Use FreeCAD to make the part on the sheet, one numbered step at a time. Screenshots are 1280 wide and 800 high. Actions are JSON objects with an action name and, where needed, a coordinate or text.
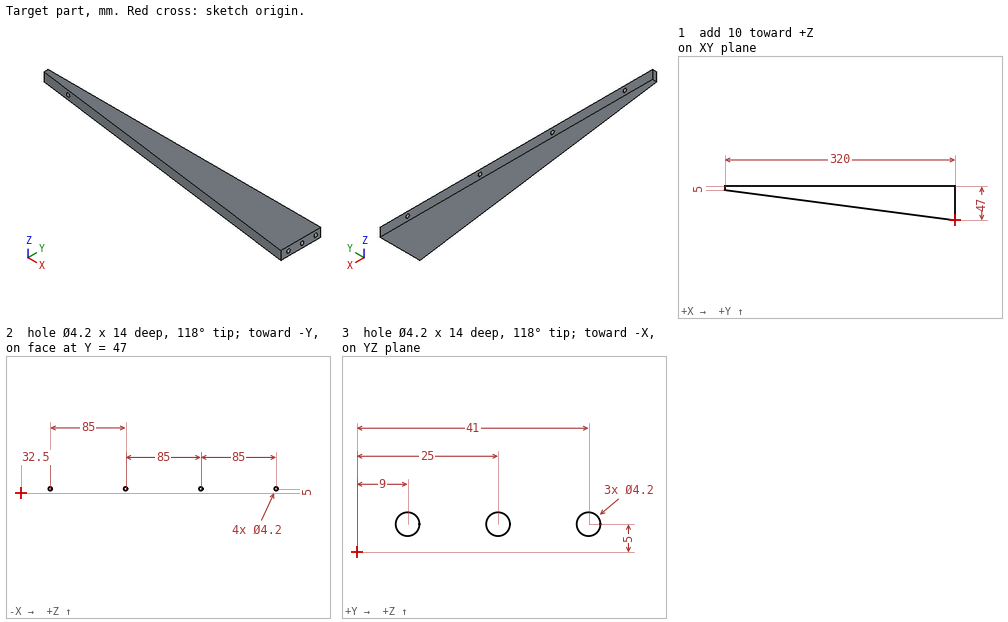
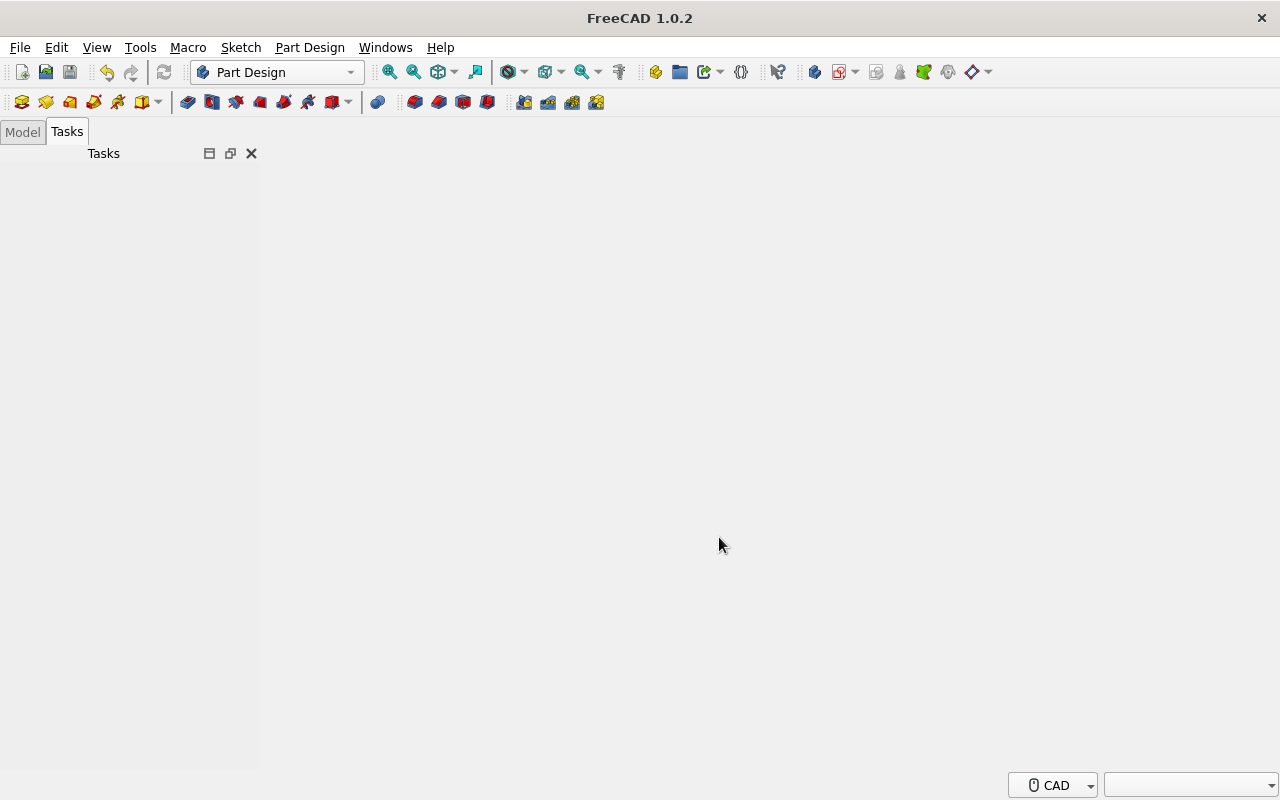
{"action": "key", "text": "ctrl+n"}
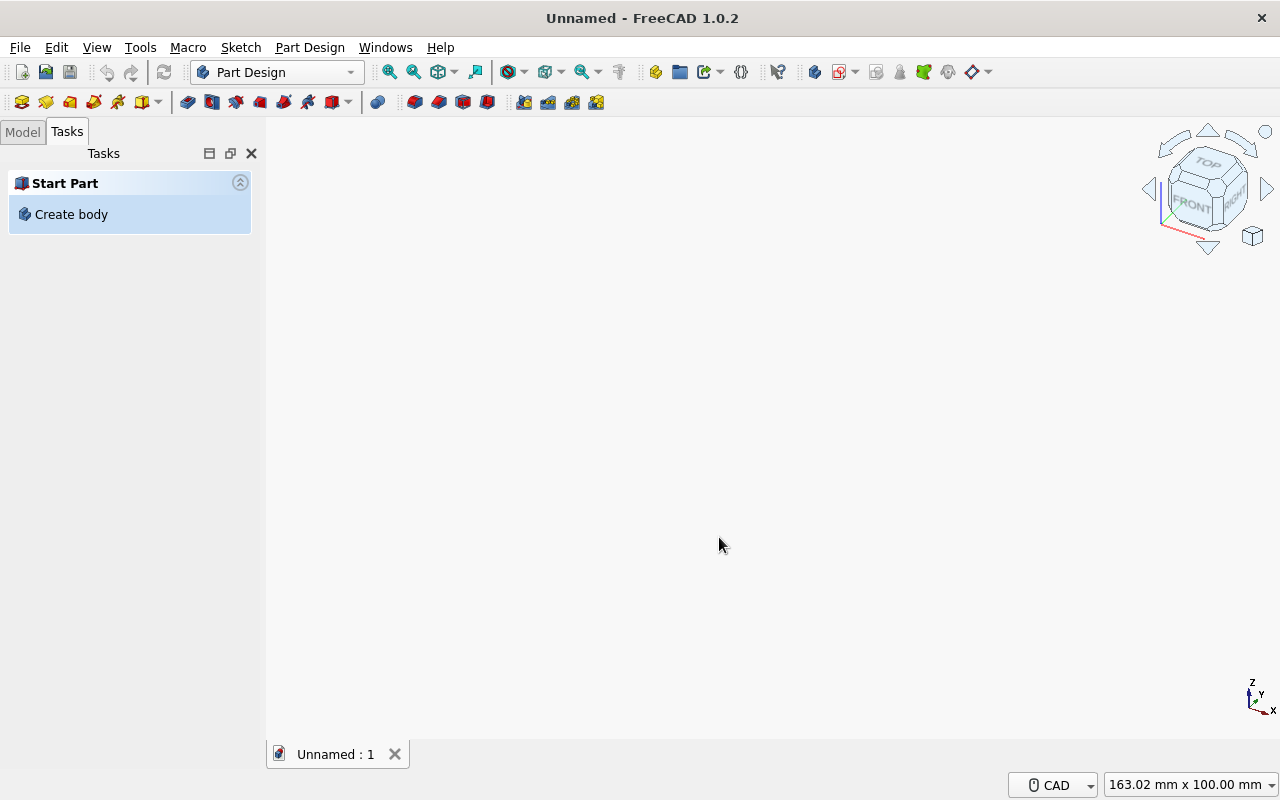
{"action": "left_click", "coordinate": [840, 72]}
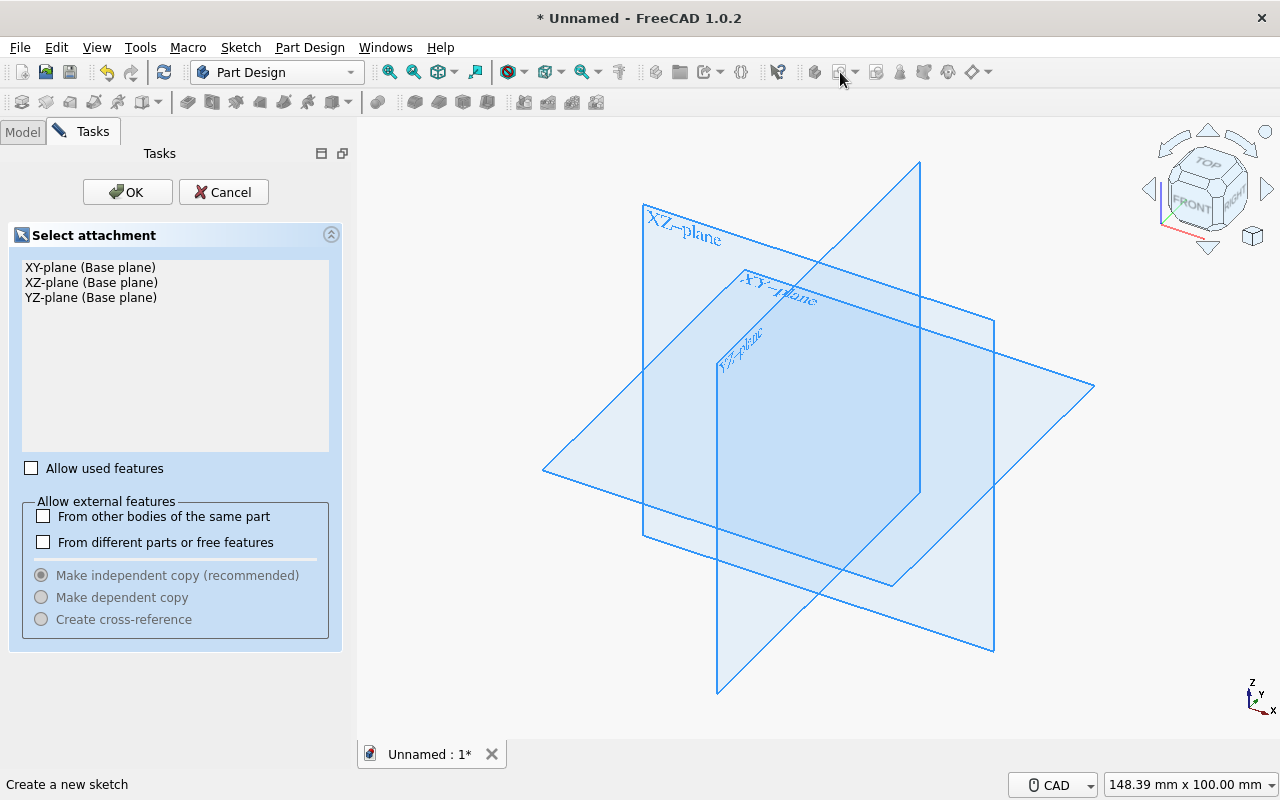
{"action": "left_click", "coordinate": [82, 268]}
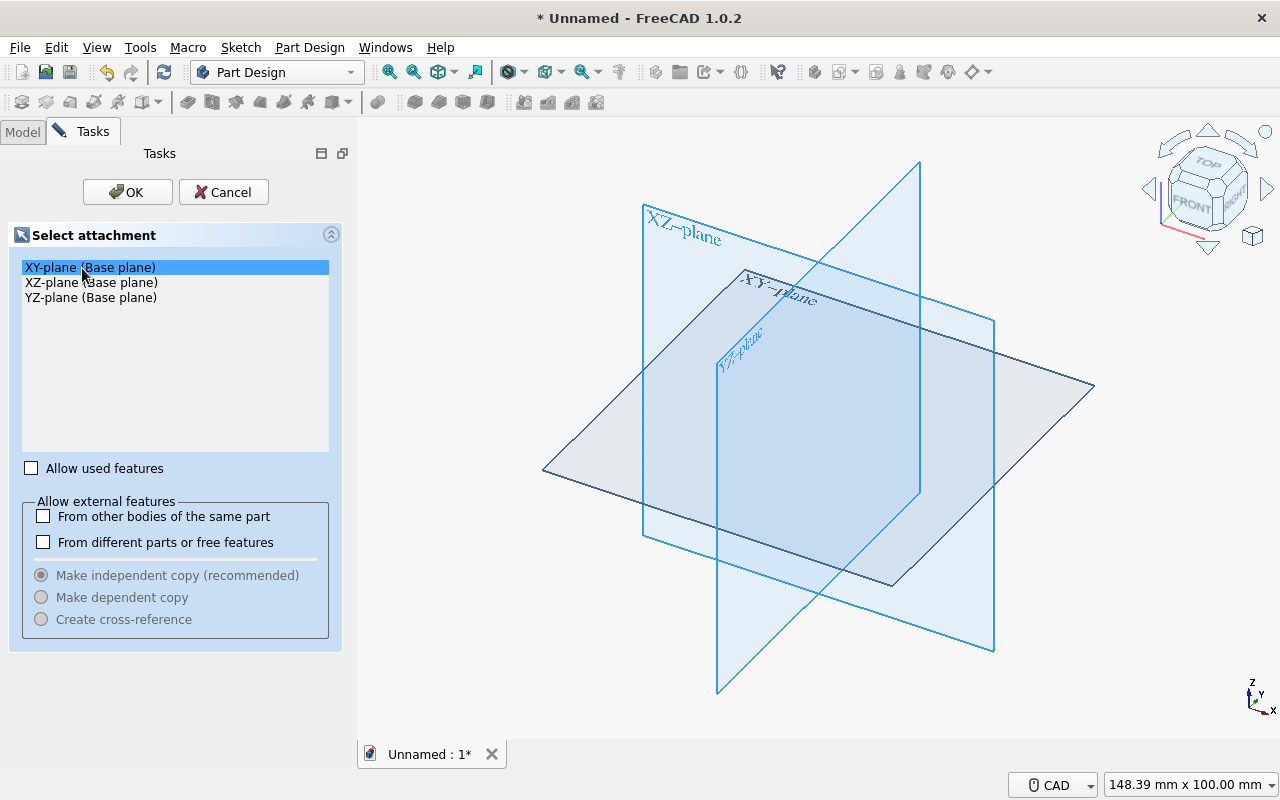
{"action": "left_click", "coordinate": [128, 192]}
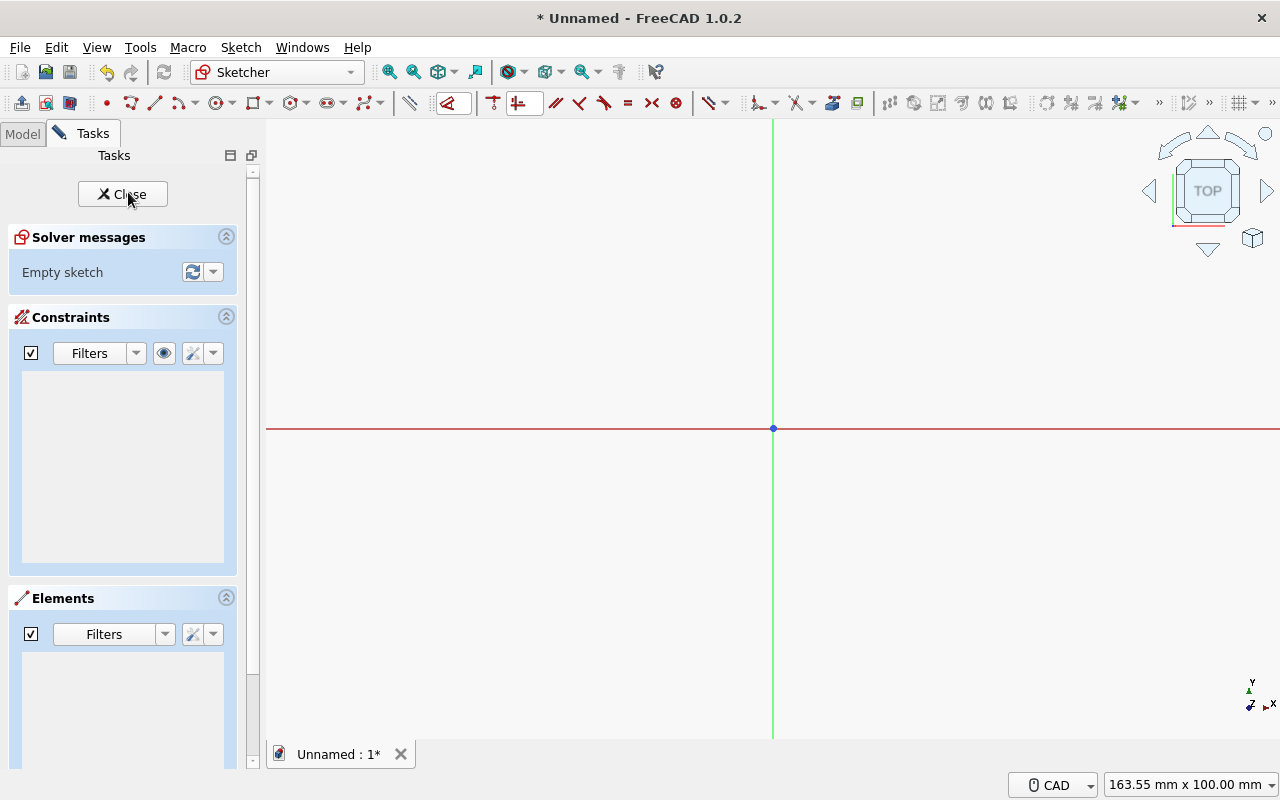
{"action": "scroll", "coordinate": [1103, 492], "scroll_direction": "down", "scroll_amount": 6}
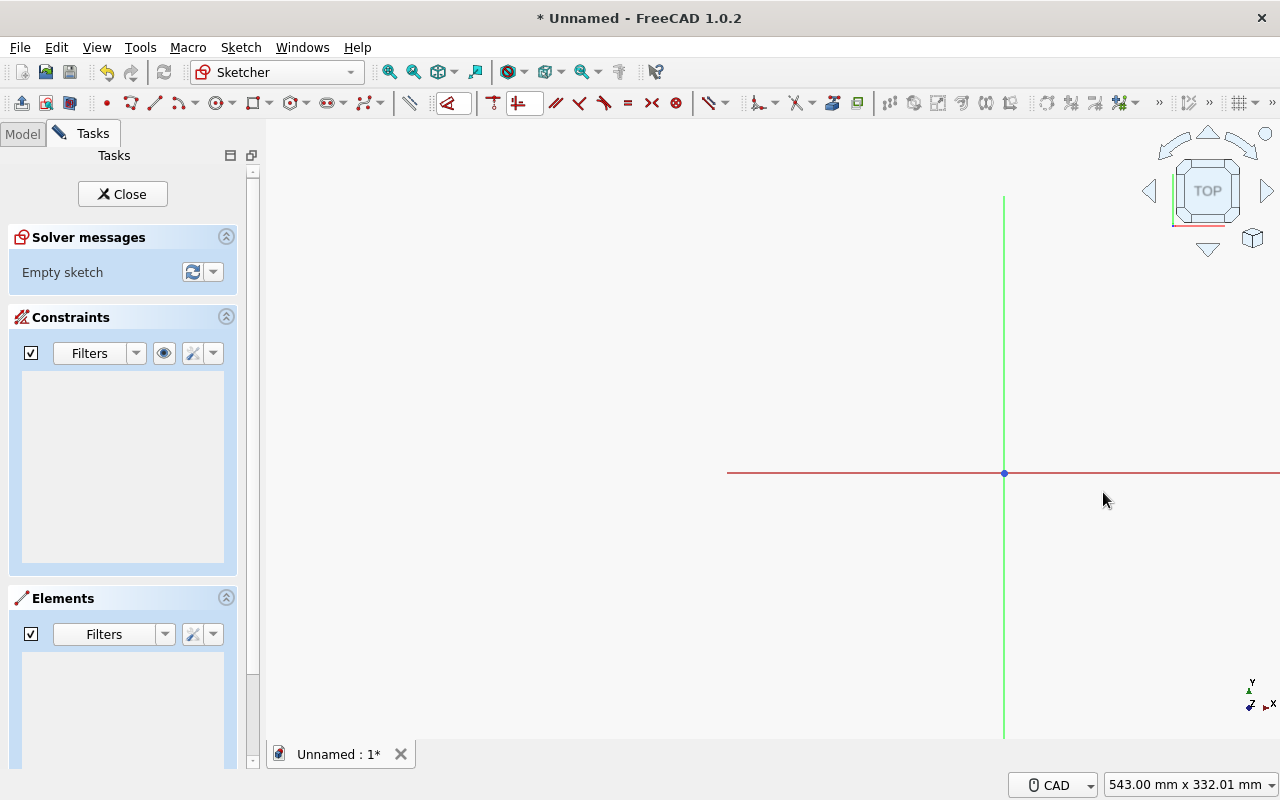
{"action": "left_click", "coordinate": [132, 104]}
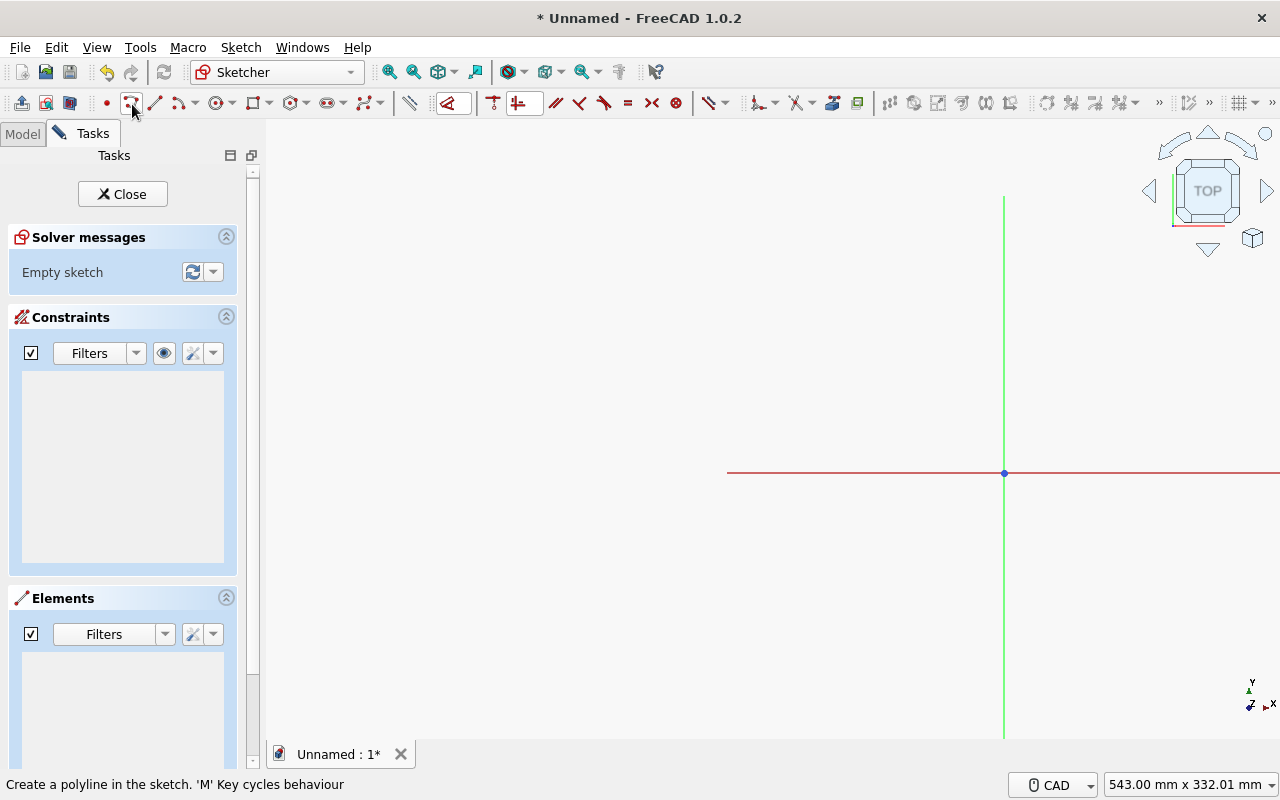
{"action": "left_click", "coordinate": [1004, 473]}
{"action": "left_click", "coordinate": [995, 386]}
{"action": "left_click", "coordinate": [407, 386]}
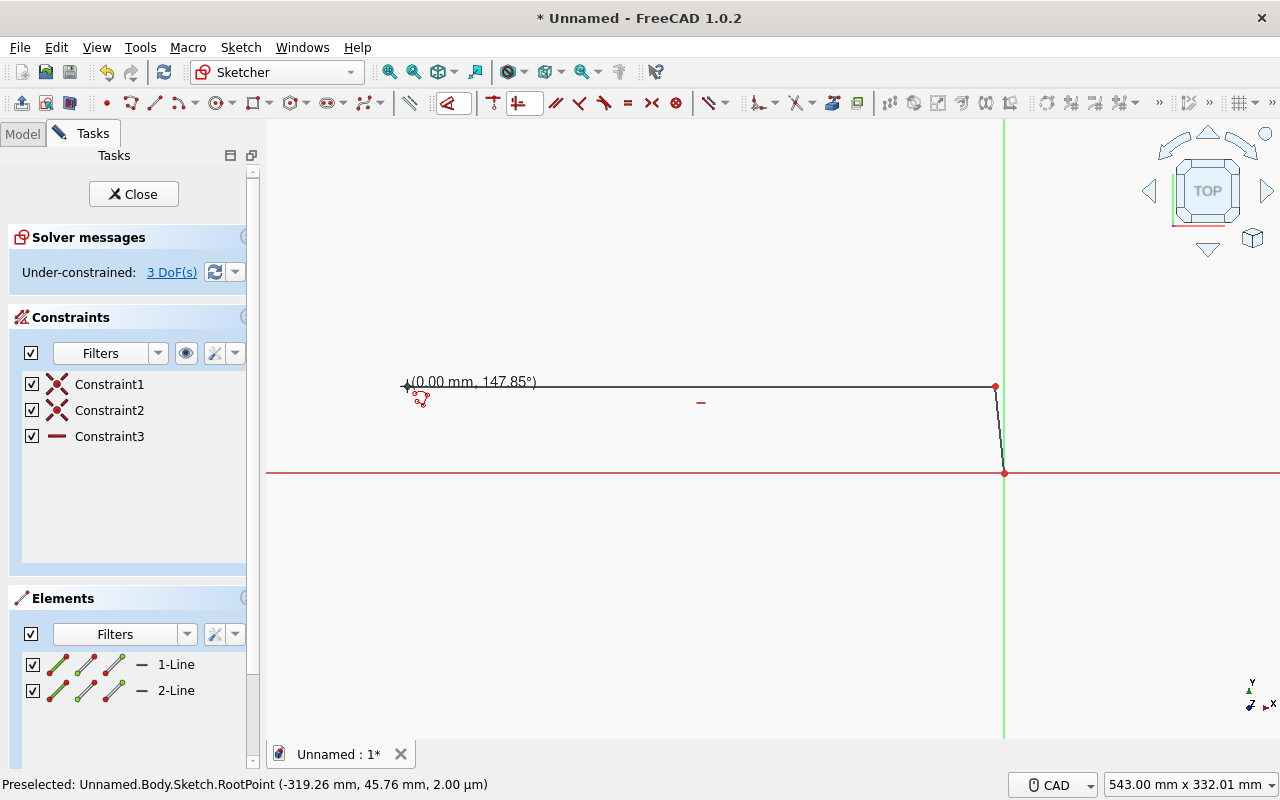
{"action": "scroll", "coordinate": [407, 395], "scroll_direction": "up", "scroll_amount": 3}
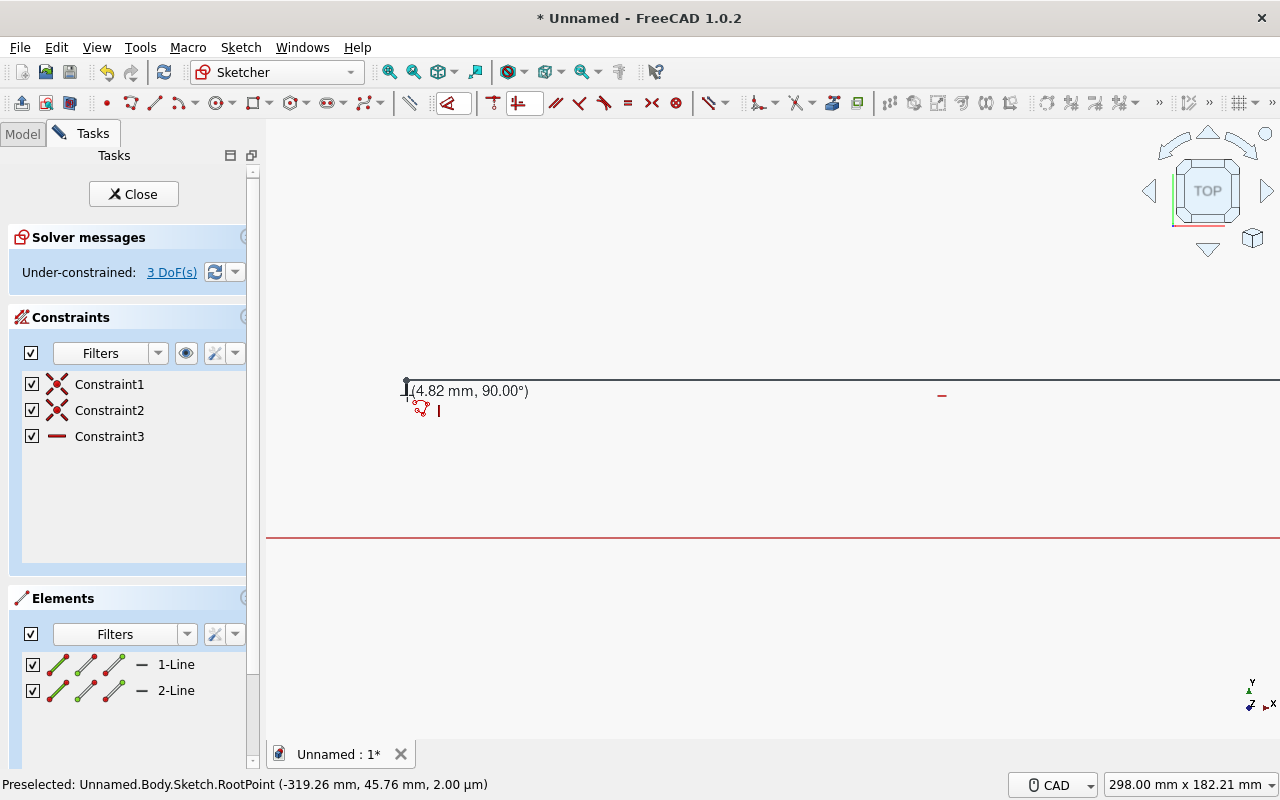
{"action": "left_click", "coordinate": [407, 395]}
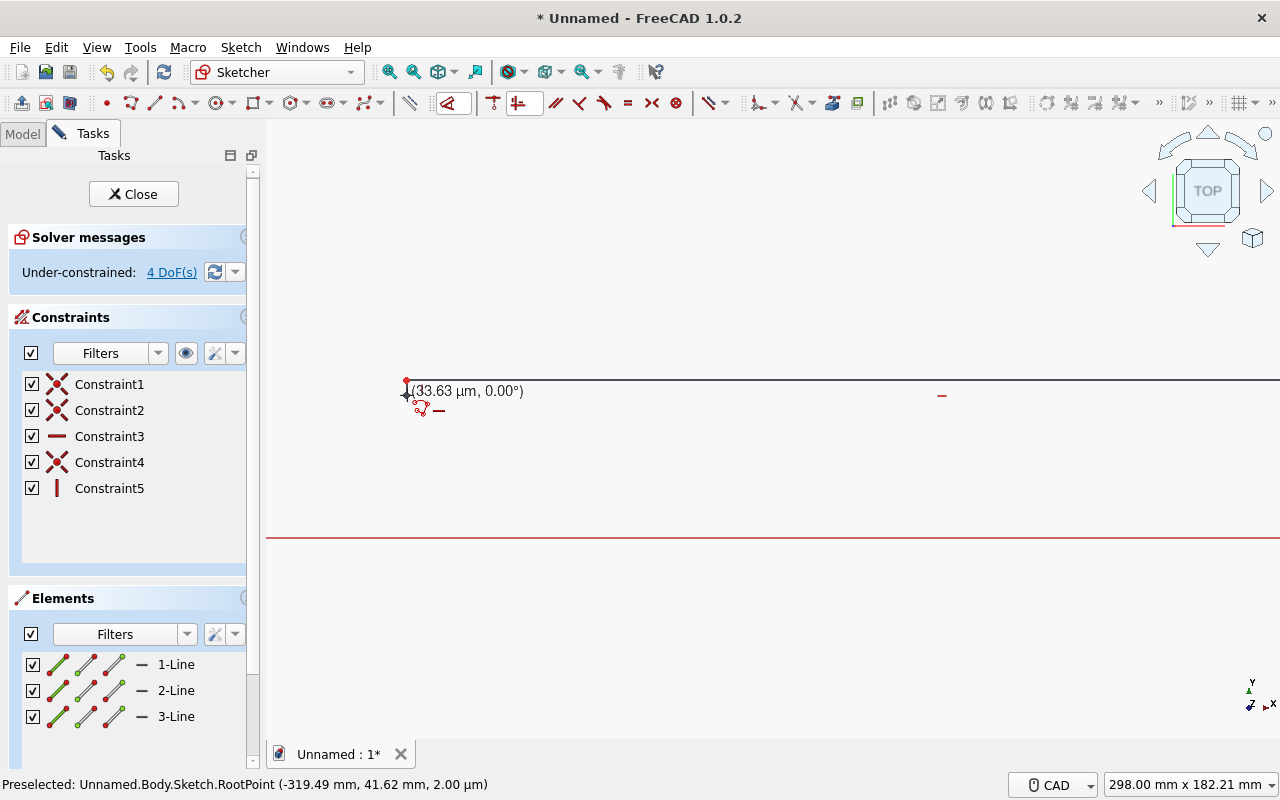
{"action": "scroll", "coordinate": [405, 394], "scroll_direction": "down", "scroll_amount": 3}